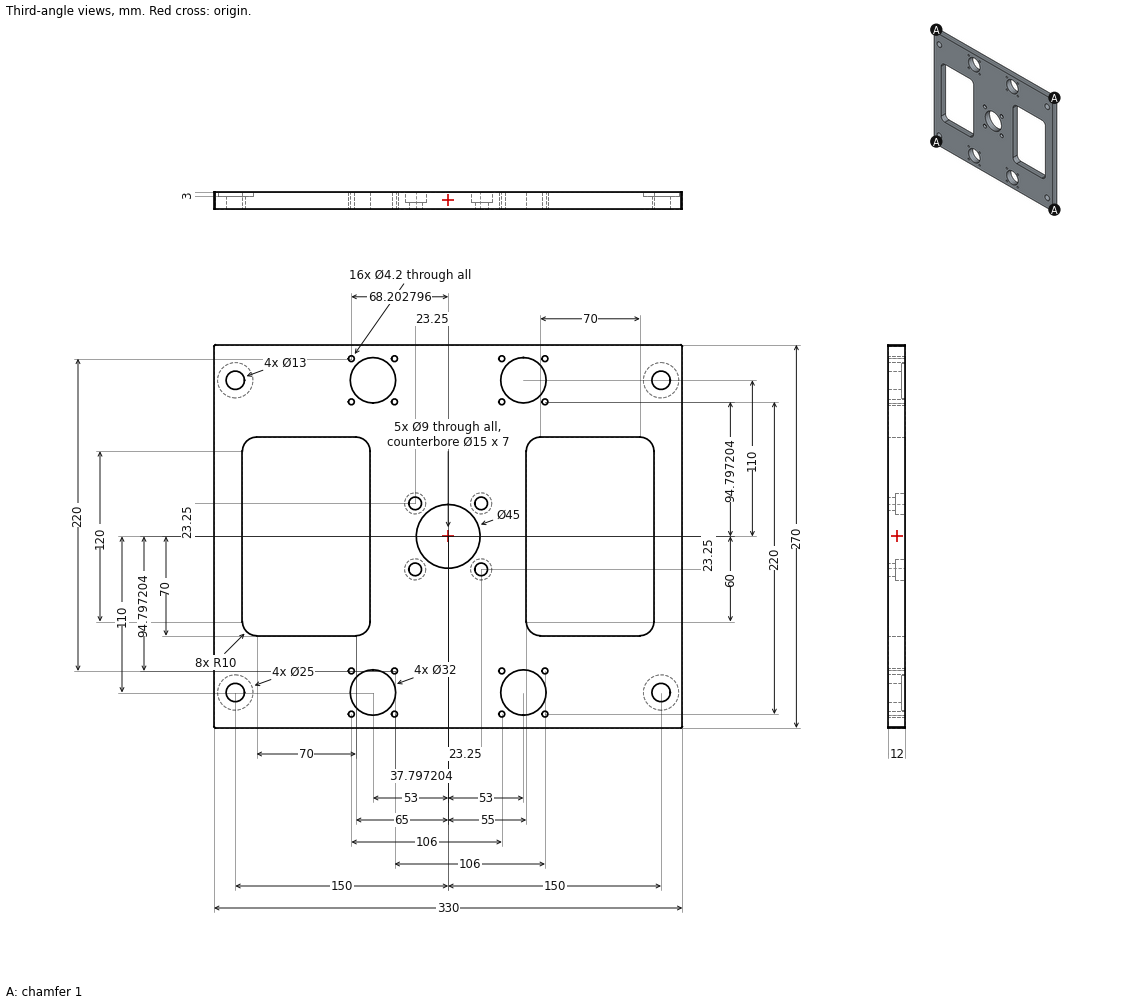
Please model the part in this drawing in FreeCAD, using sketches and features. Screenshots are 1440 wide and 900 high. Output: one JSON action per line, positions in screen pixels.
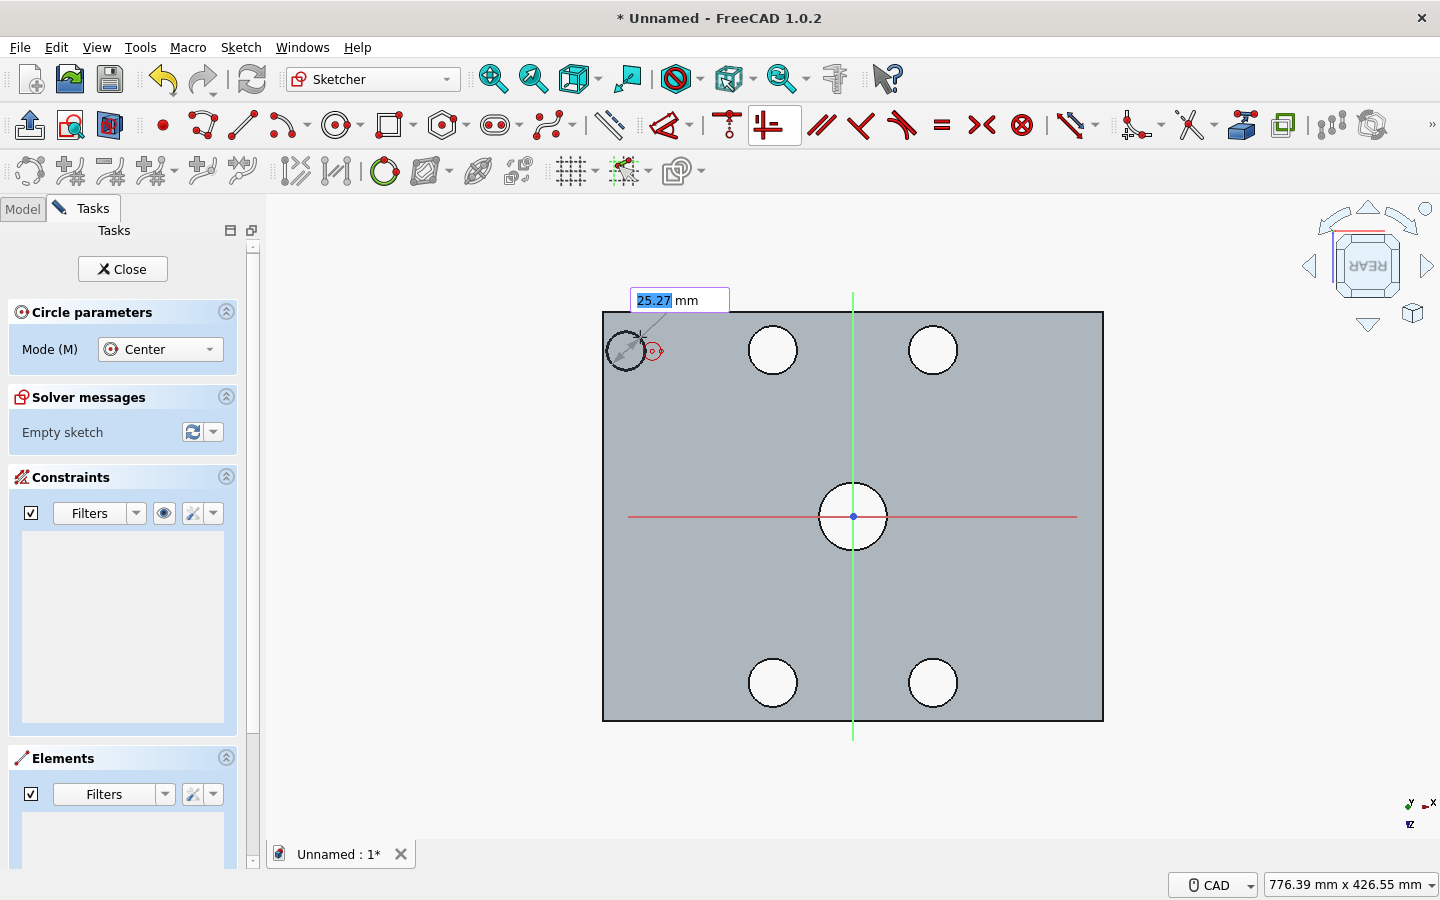
{"action": "type", "text": "25"}
{"action": "key", "text": "Return"}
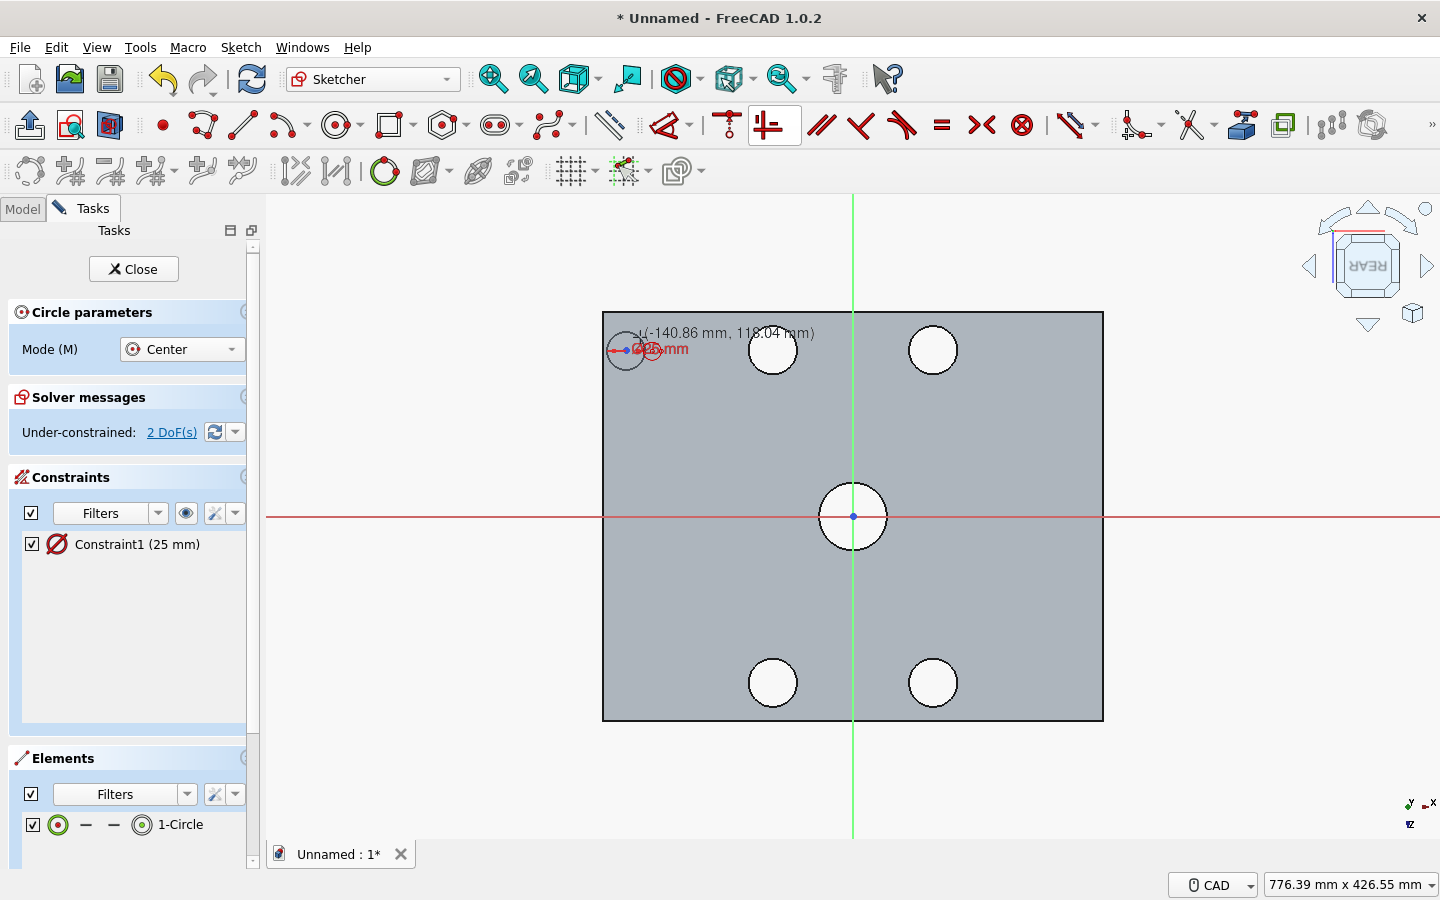
{"action": "left_click", "coordinate": [1080, 350]}
{"action": "mouse_move", "coordinate": [1093, 337]}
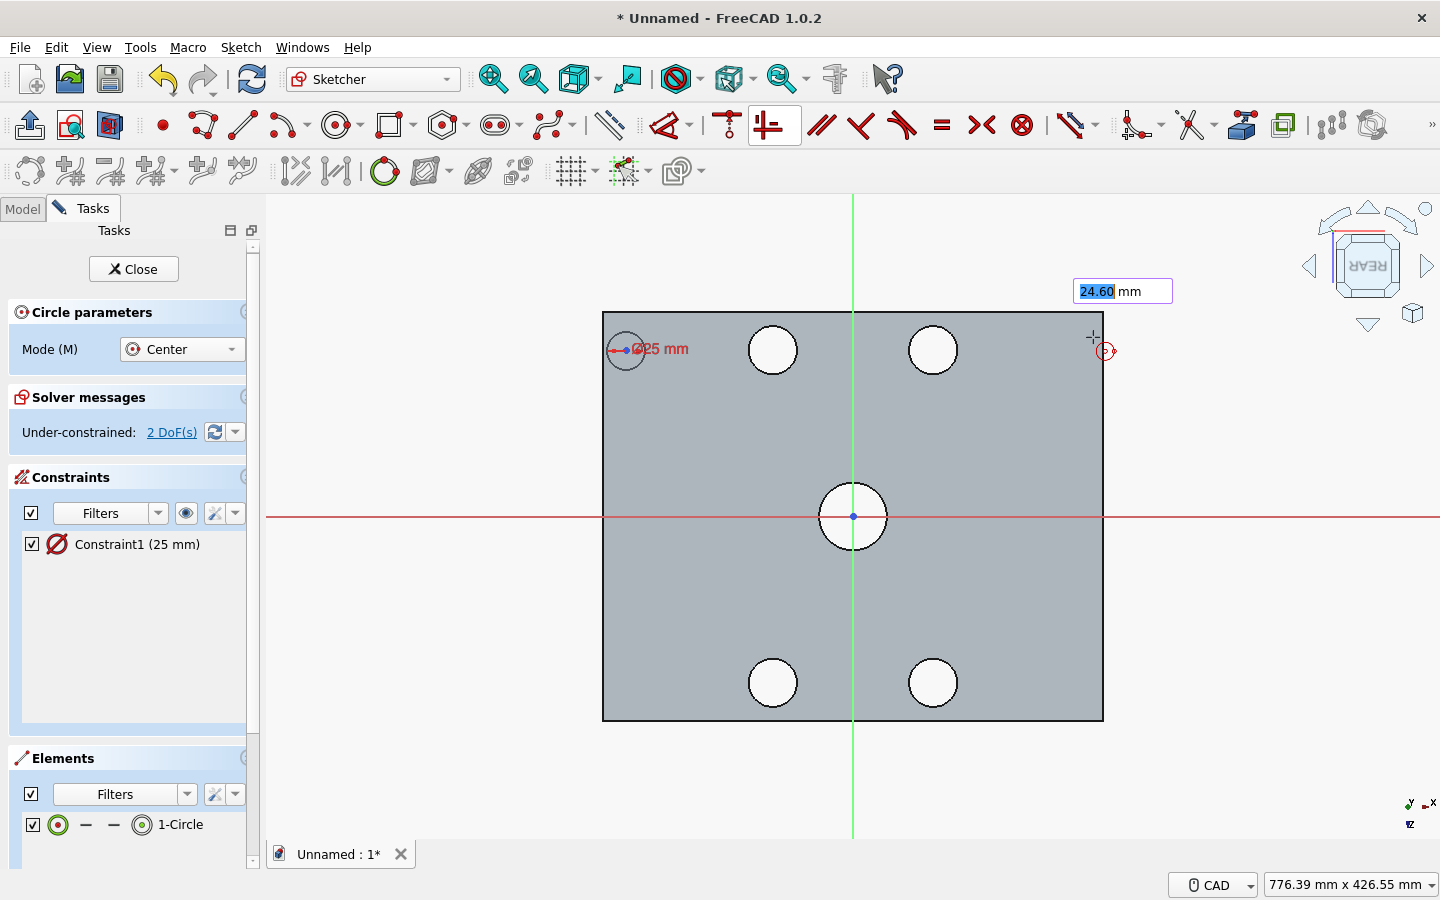
{"action": "type", "text": "25"}
{"action": "key", "text": "Return"}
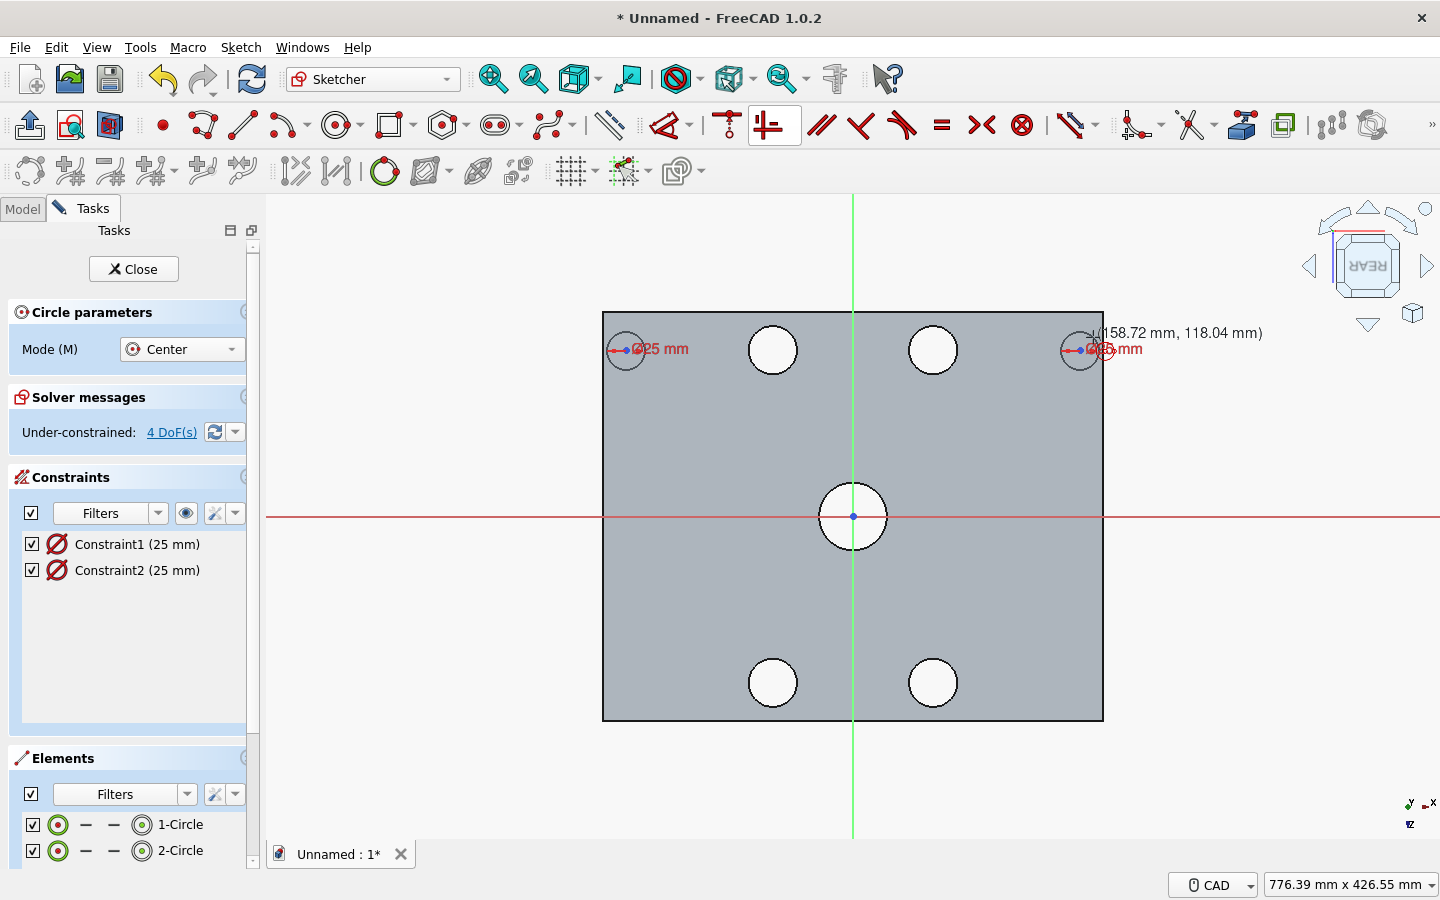
{"action": "left_click", "coordinate": [1080, 683]}
{"action": "mouse_move", "coordinate": [1093, 669]}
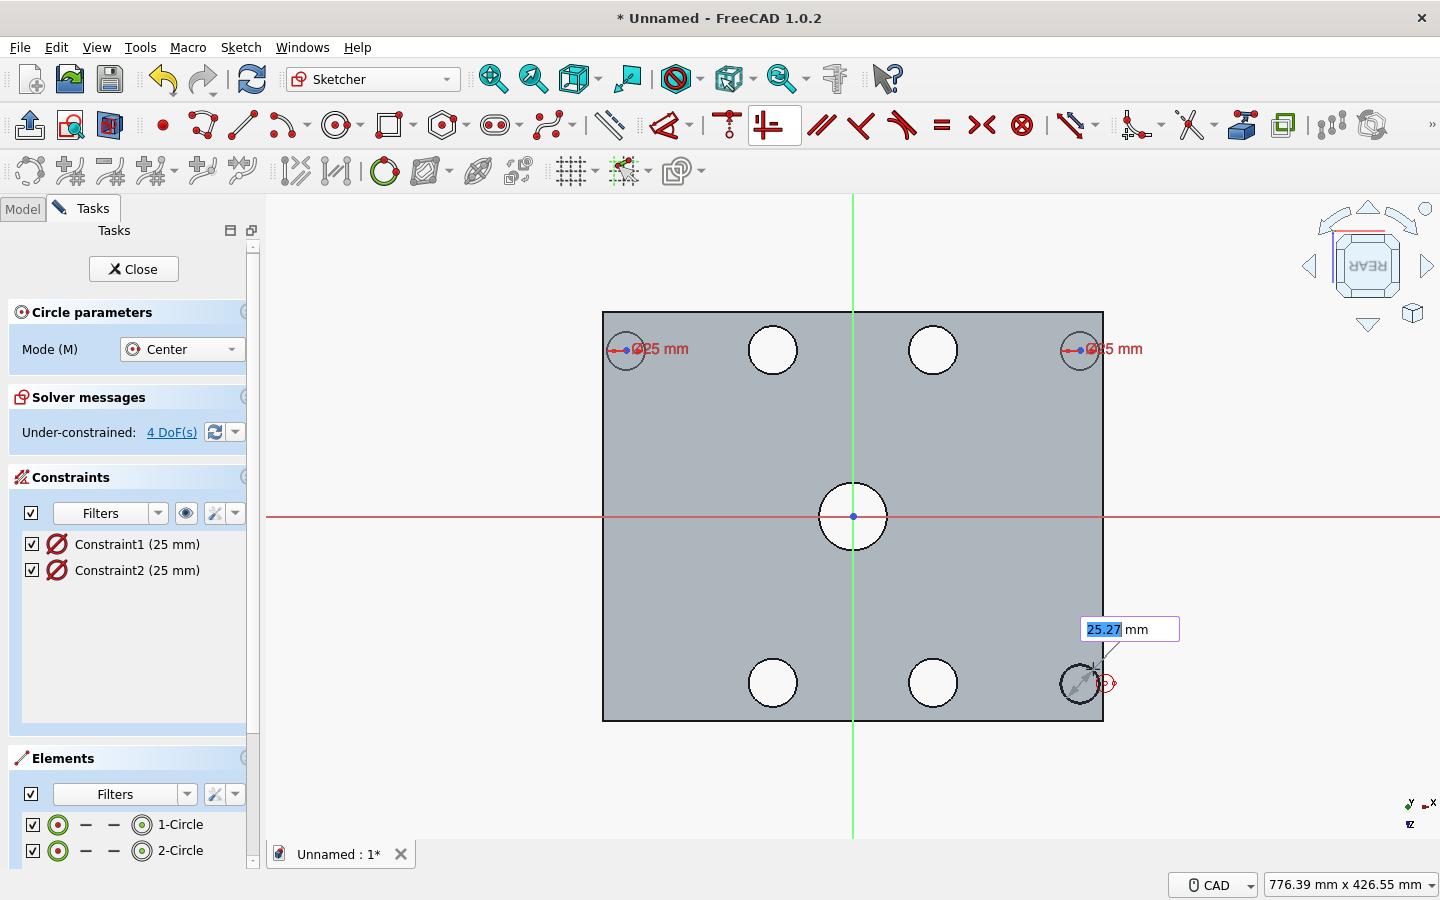
{"action": "type", "text": "25"}
{"action": "key", "text": "Return"}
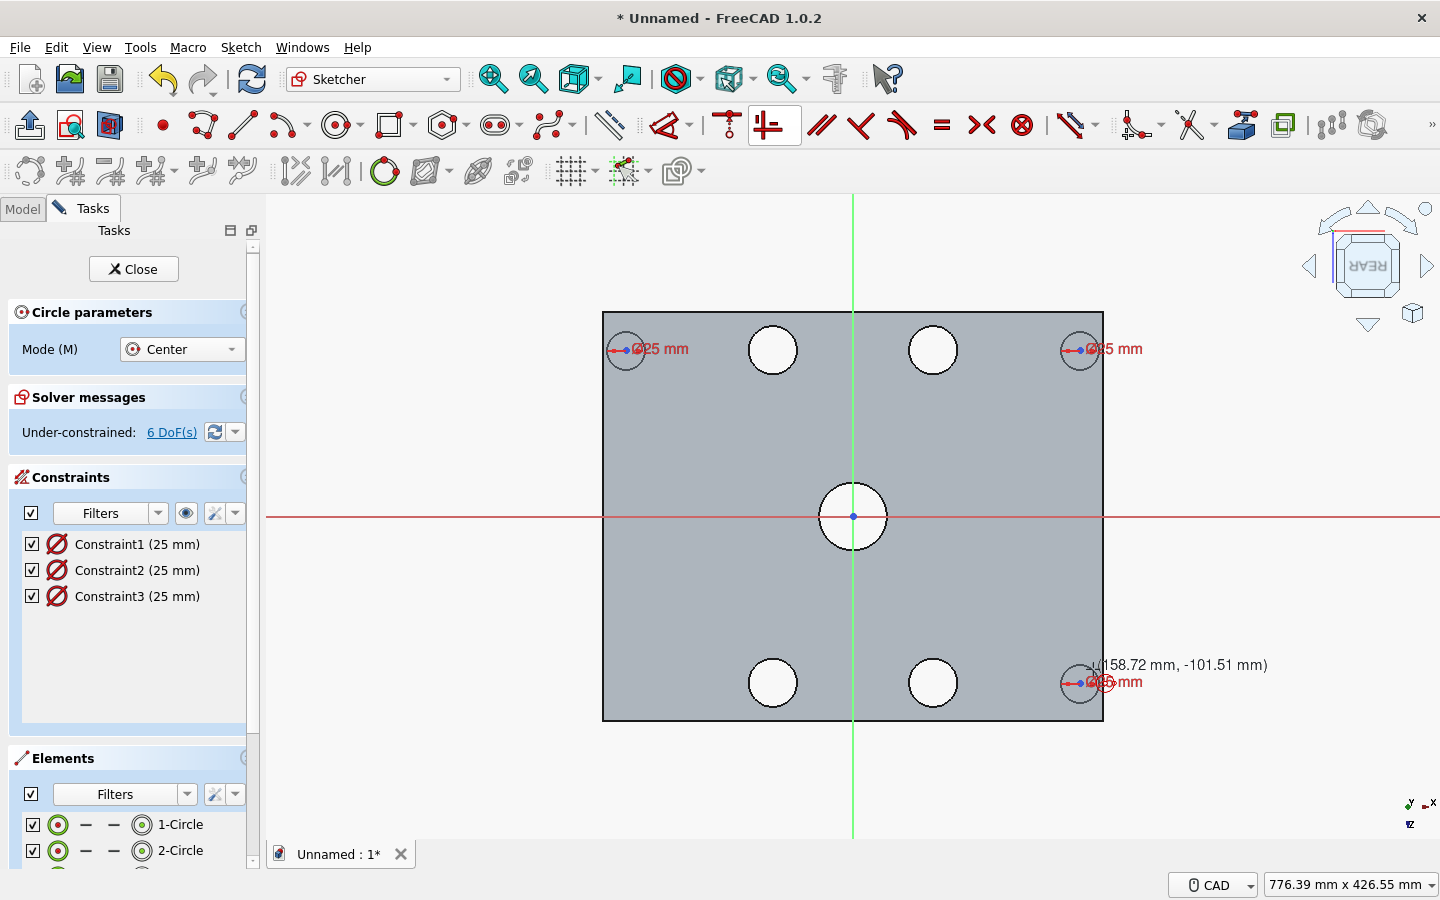
{"action": "left_click", "coordinate": [626, 683]}
{"action": "mouse_move", "coordinate": [640, 669]}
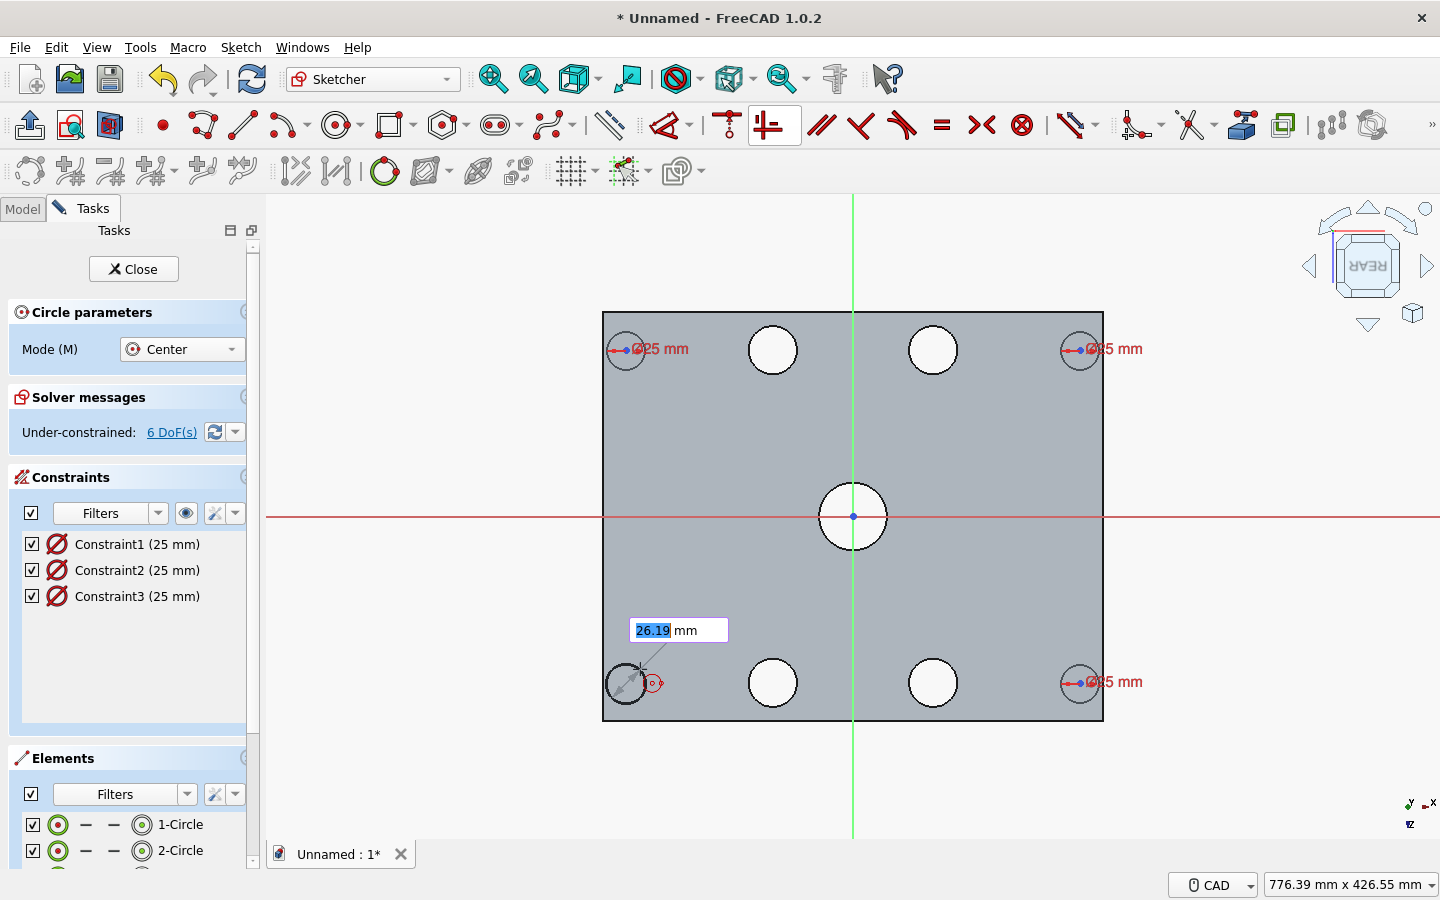
{"action": "type", "text": "25"}
{"action": "key", "text": "Return"}
{"action": "key", "text": "Escape"}